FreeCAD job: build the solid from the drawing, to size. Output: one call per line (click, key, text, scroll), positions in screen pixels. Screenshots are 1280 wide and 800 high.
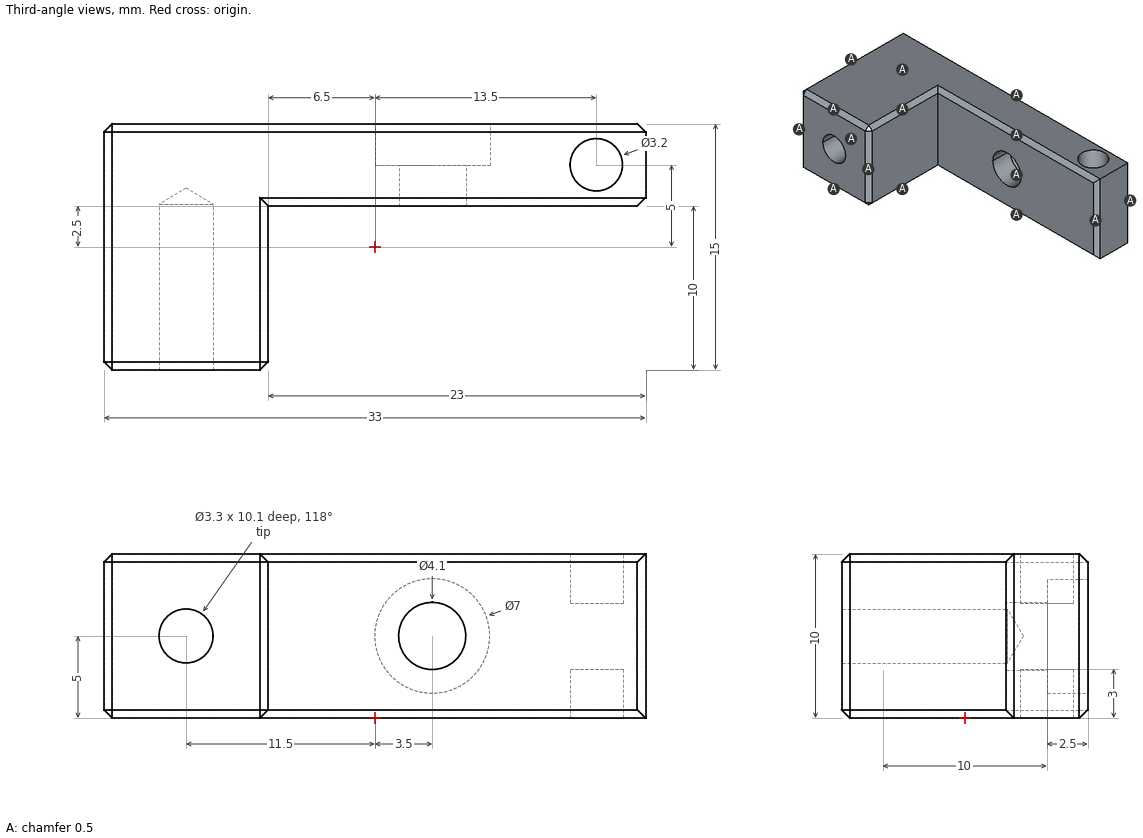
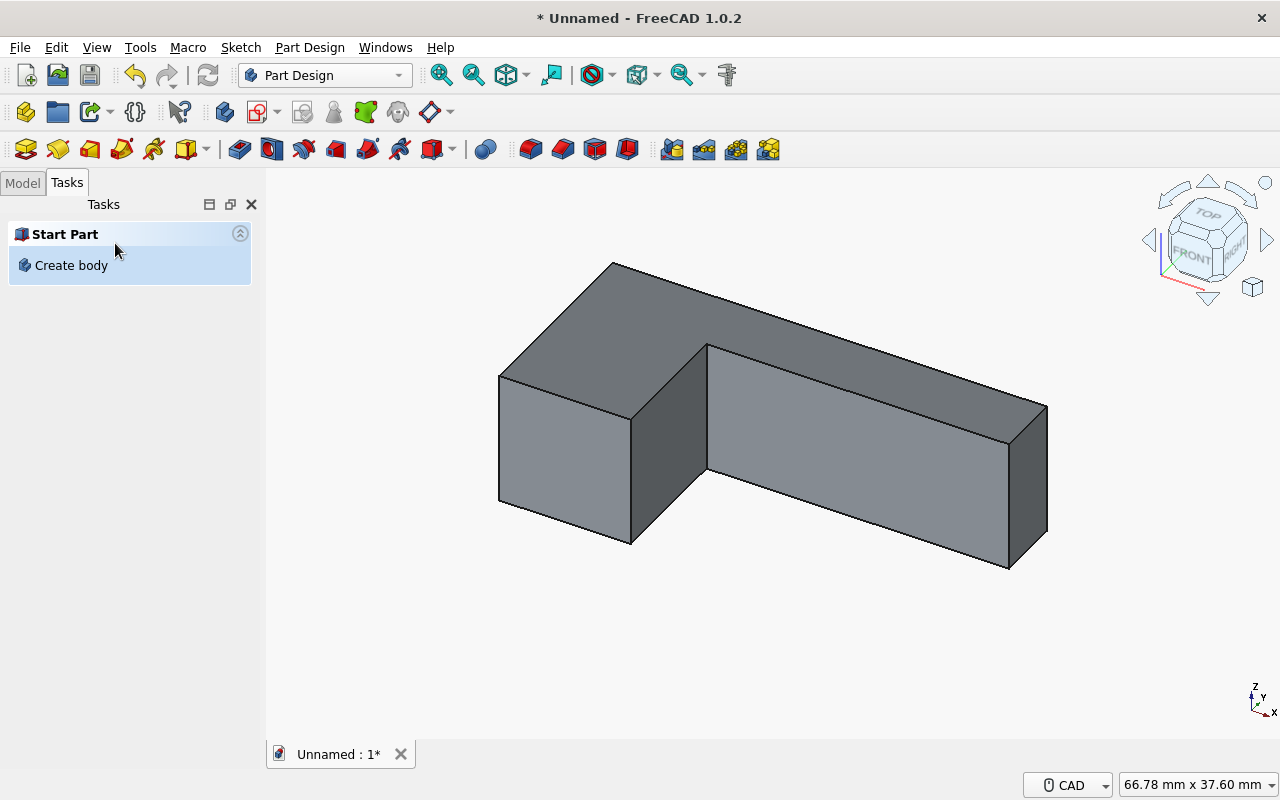
click(565, 459)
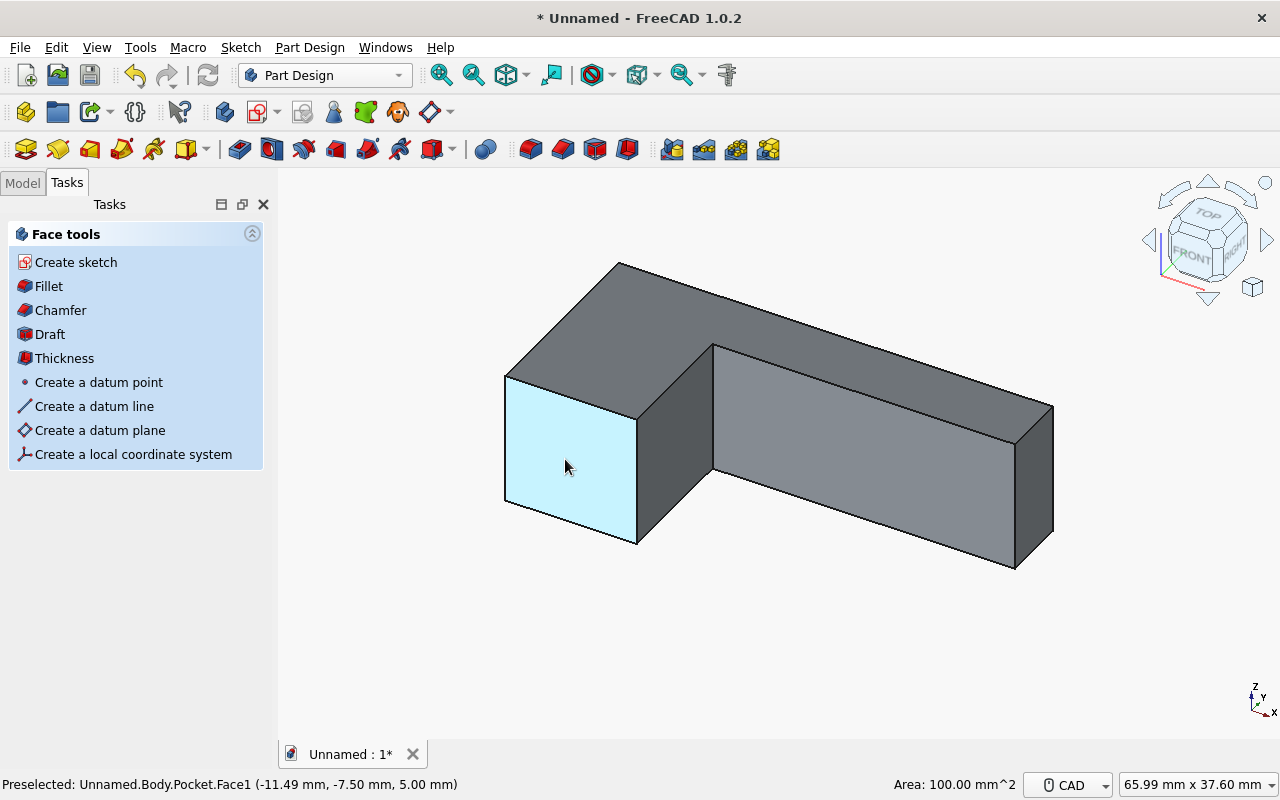
click(258, 112)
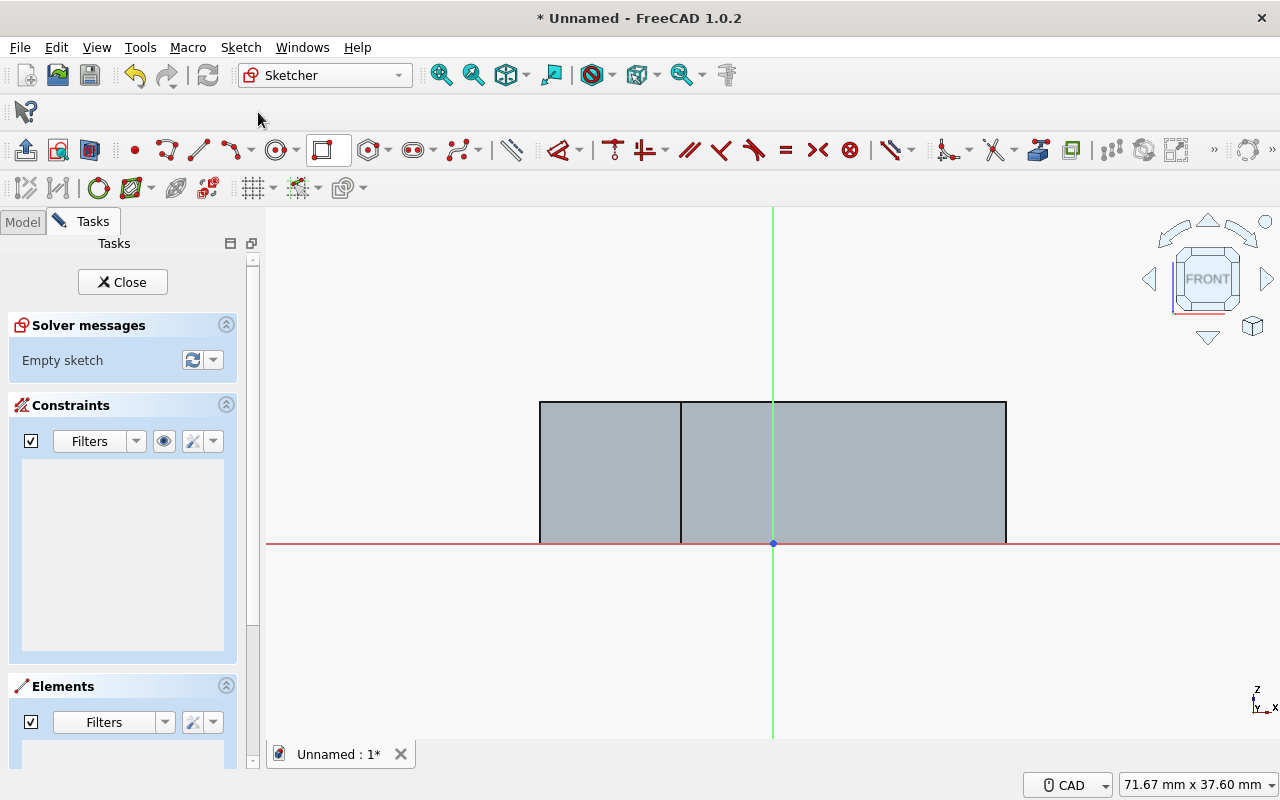
scroll(596, 473, up, 10)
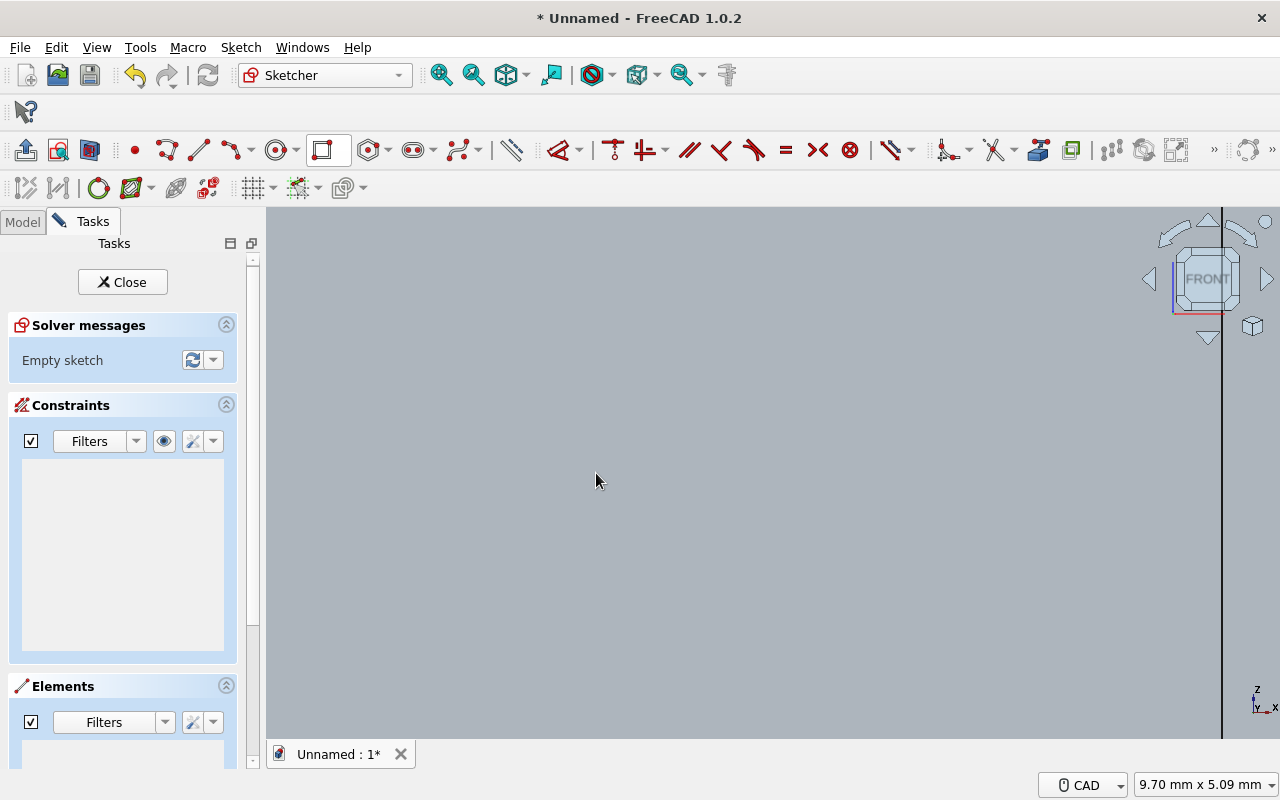
click(276, 150)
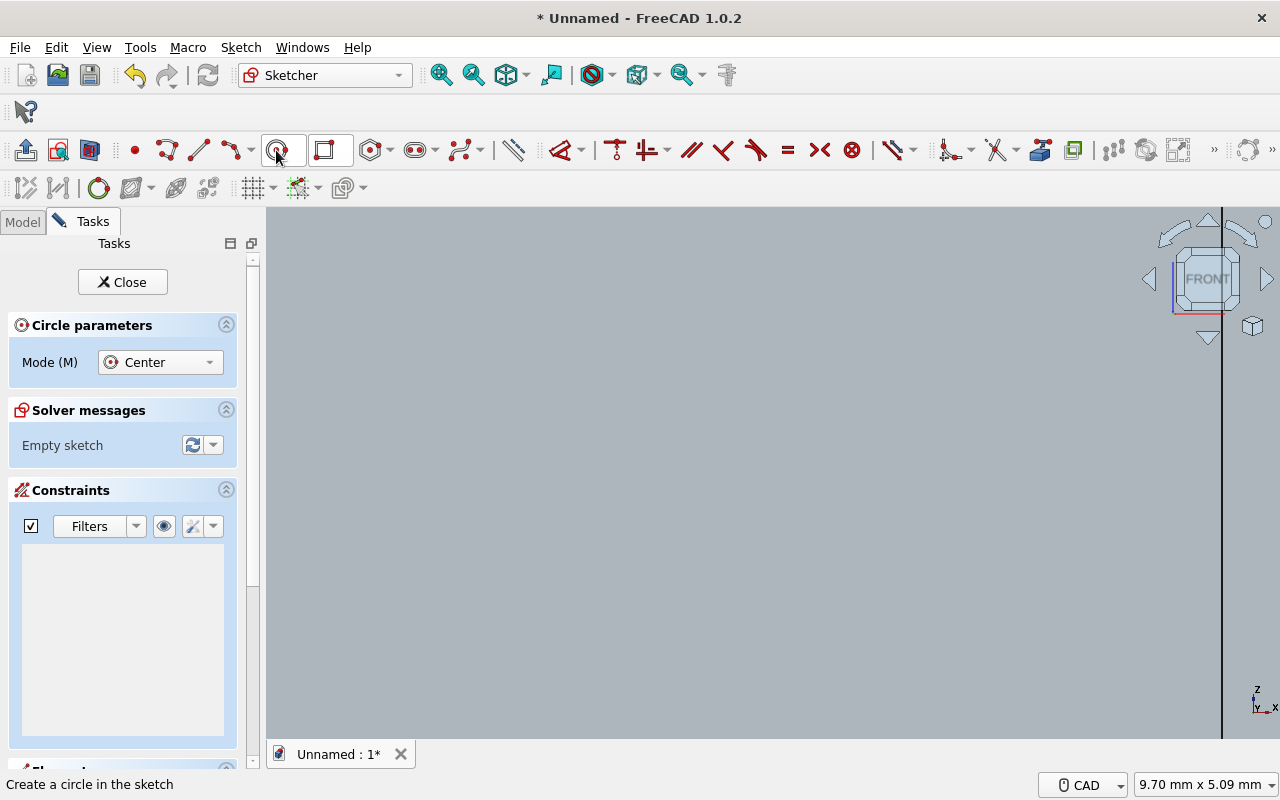
click(700, 470)
move(822, 348)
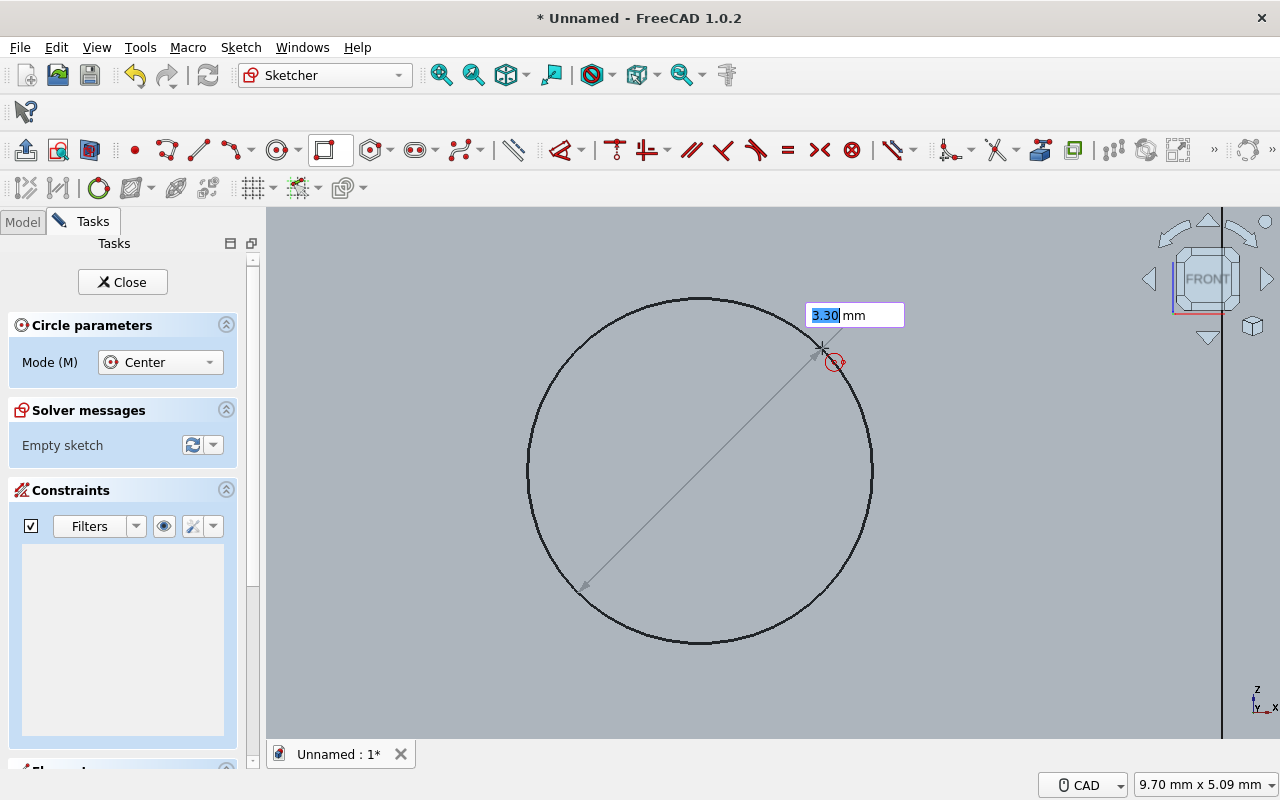
text(3.3)
key(Return)
key(Escape)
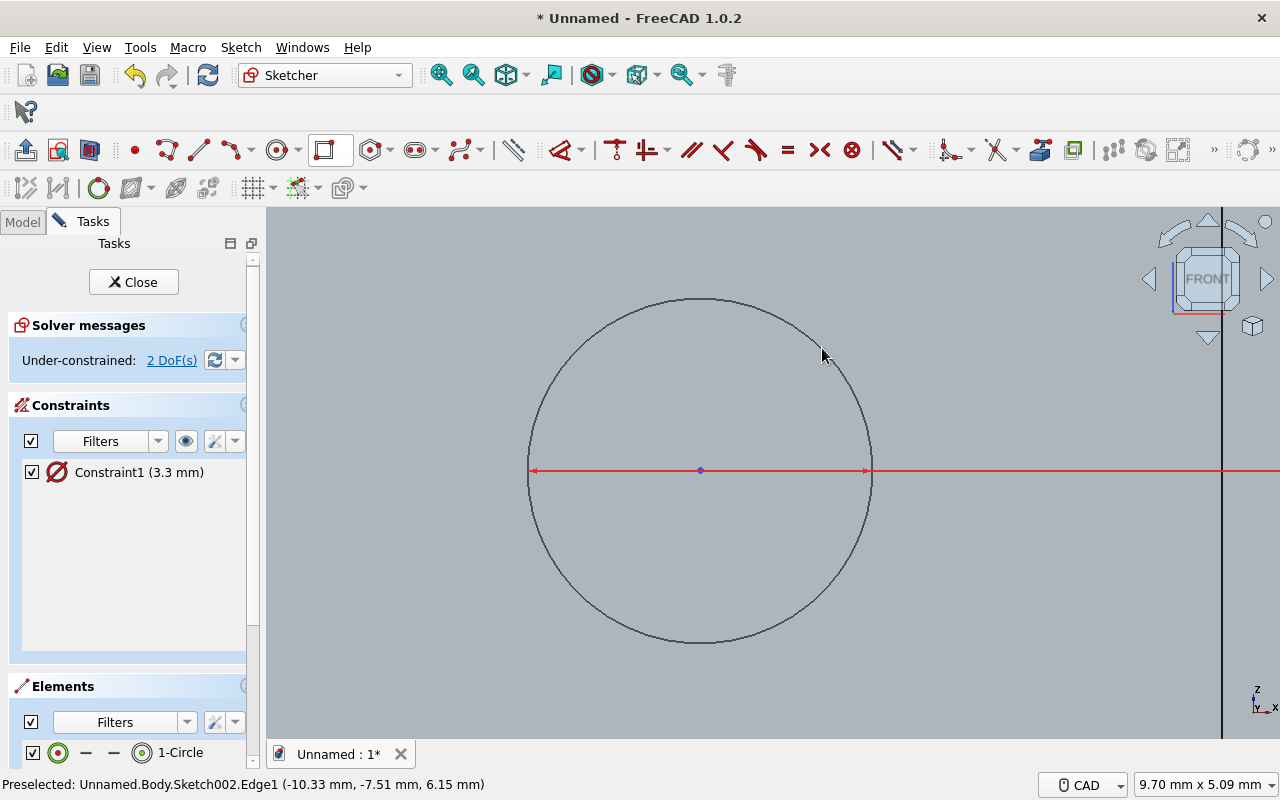
click(700, 471)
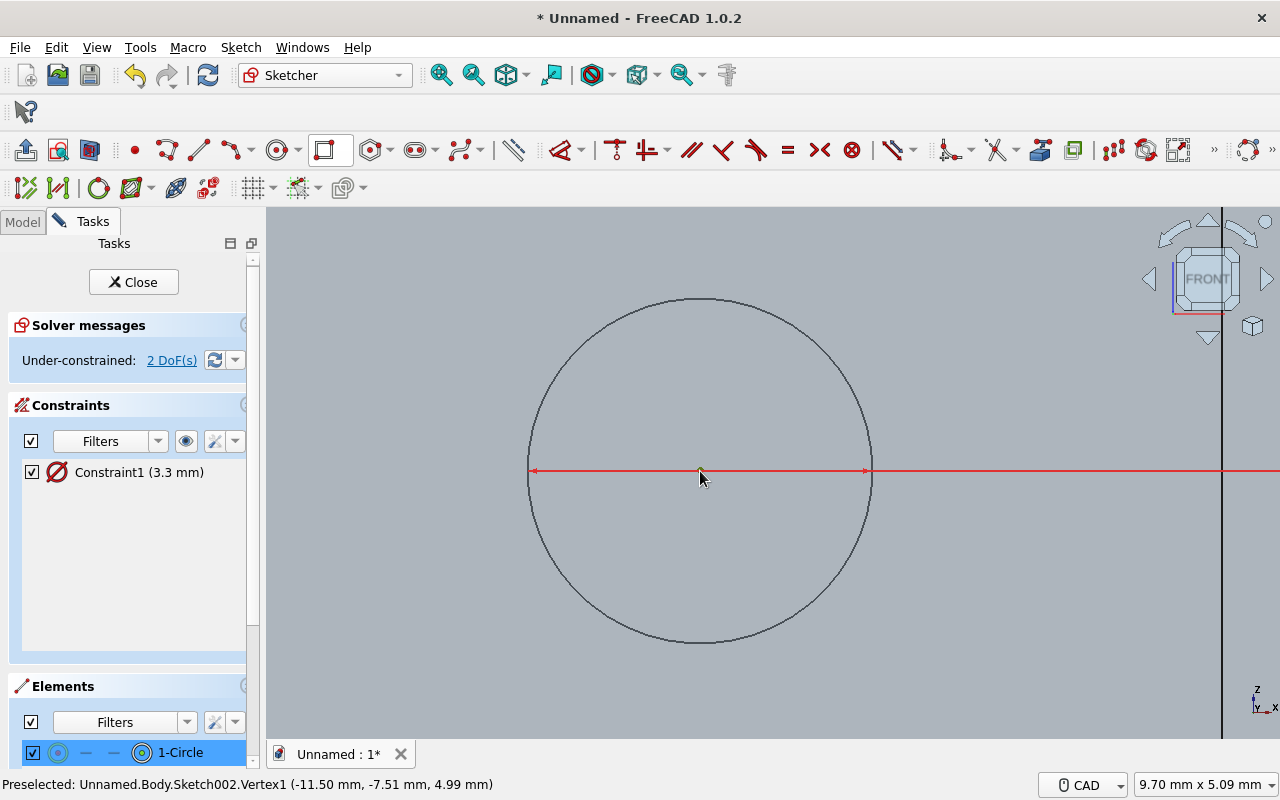
click(584, 150)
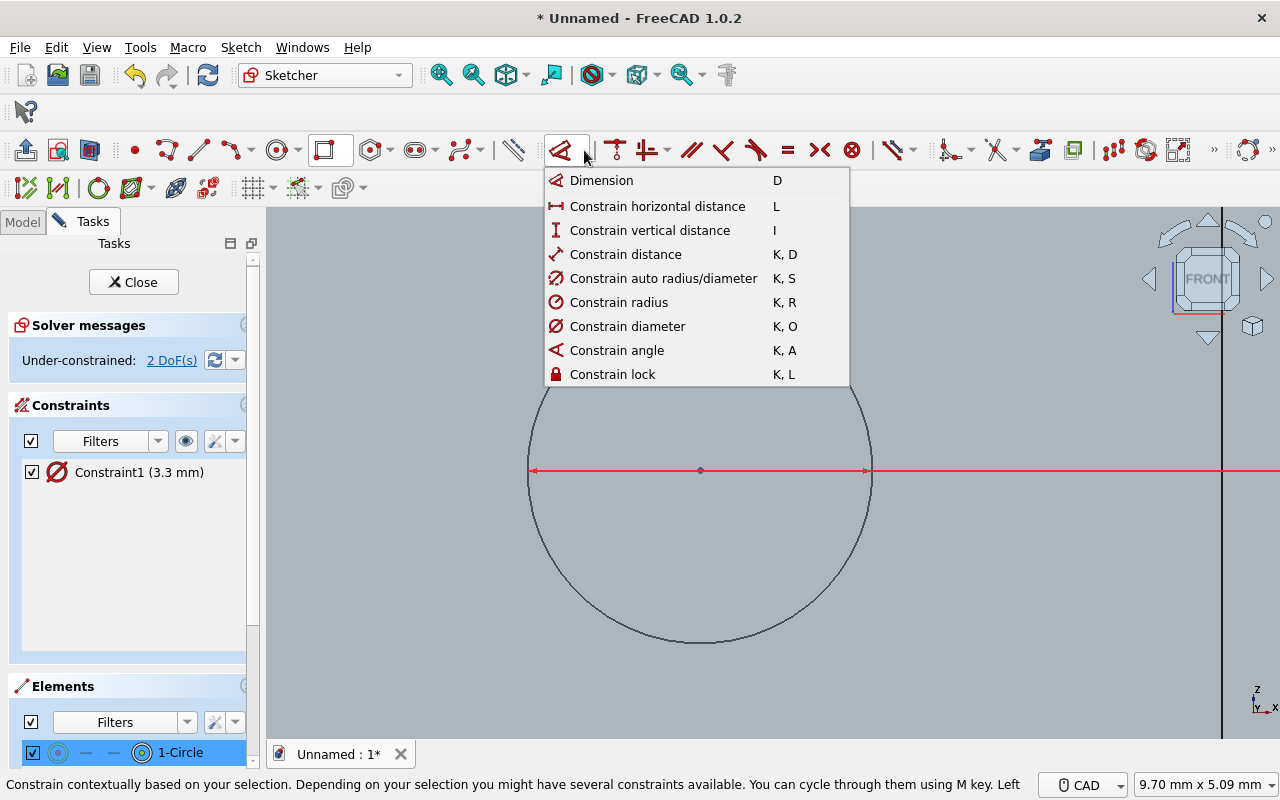
click(697, 230)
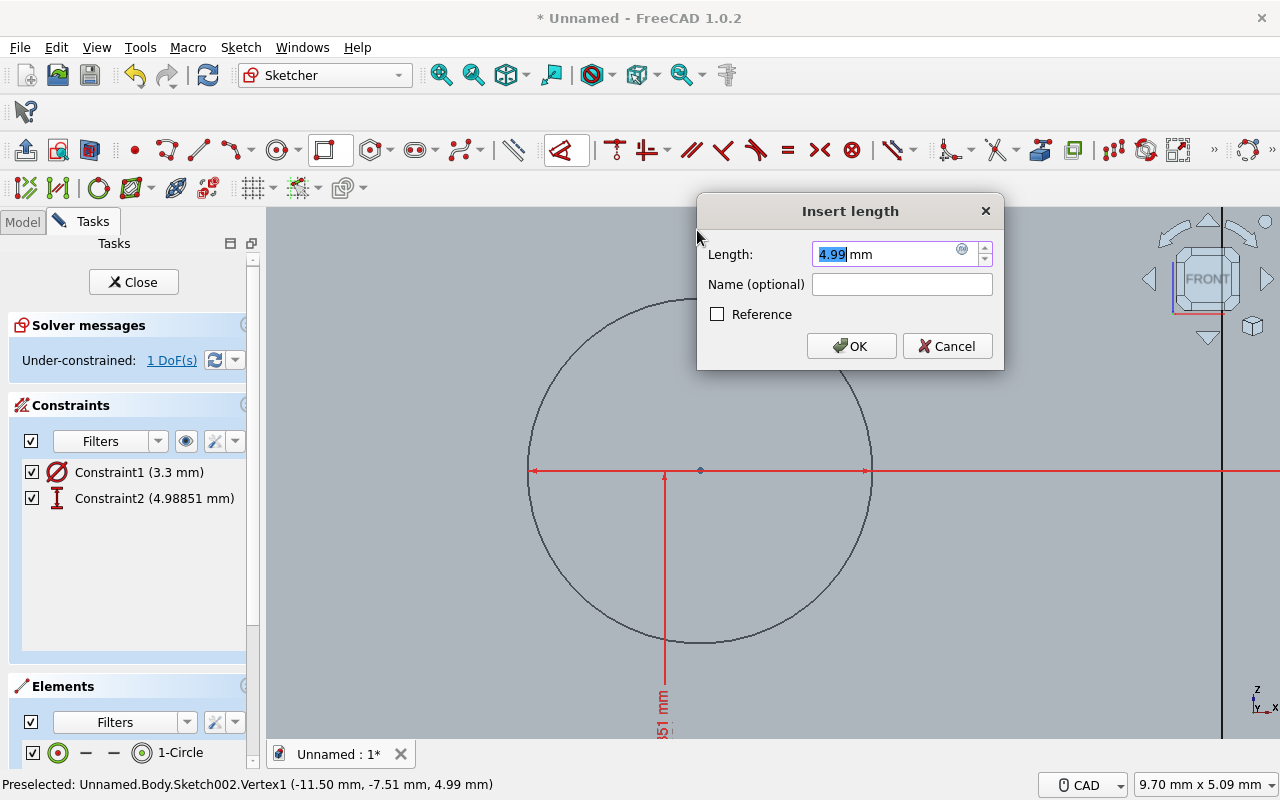
text(5)
key(Return)